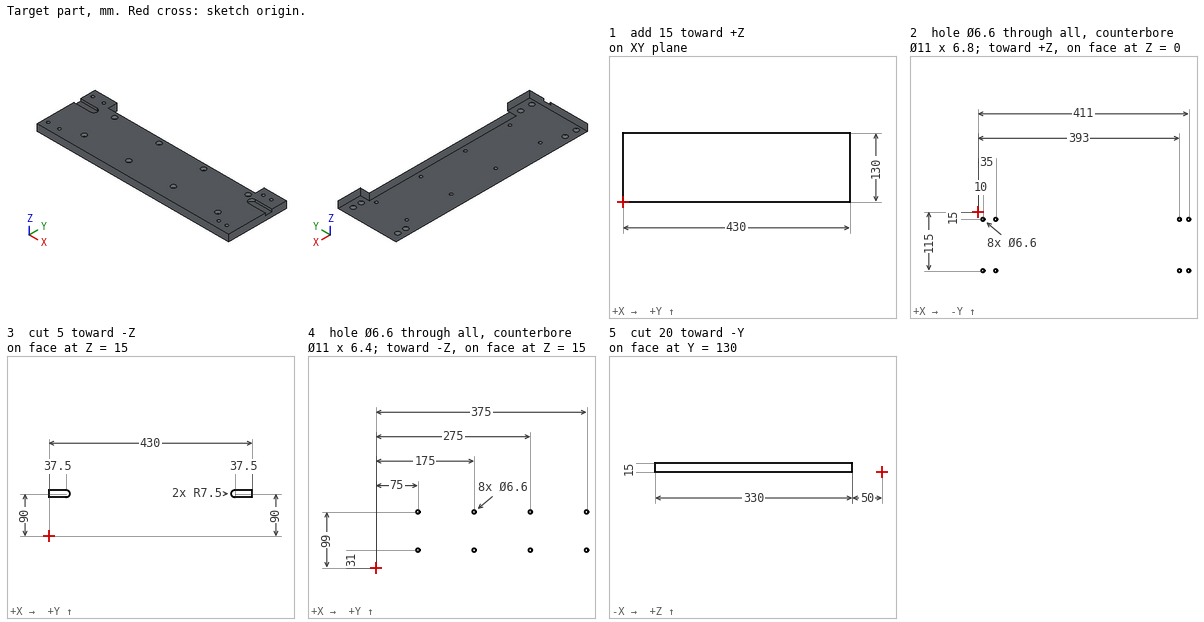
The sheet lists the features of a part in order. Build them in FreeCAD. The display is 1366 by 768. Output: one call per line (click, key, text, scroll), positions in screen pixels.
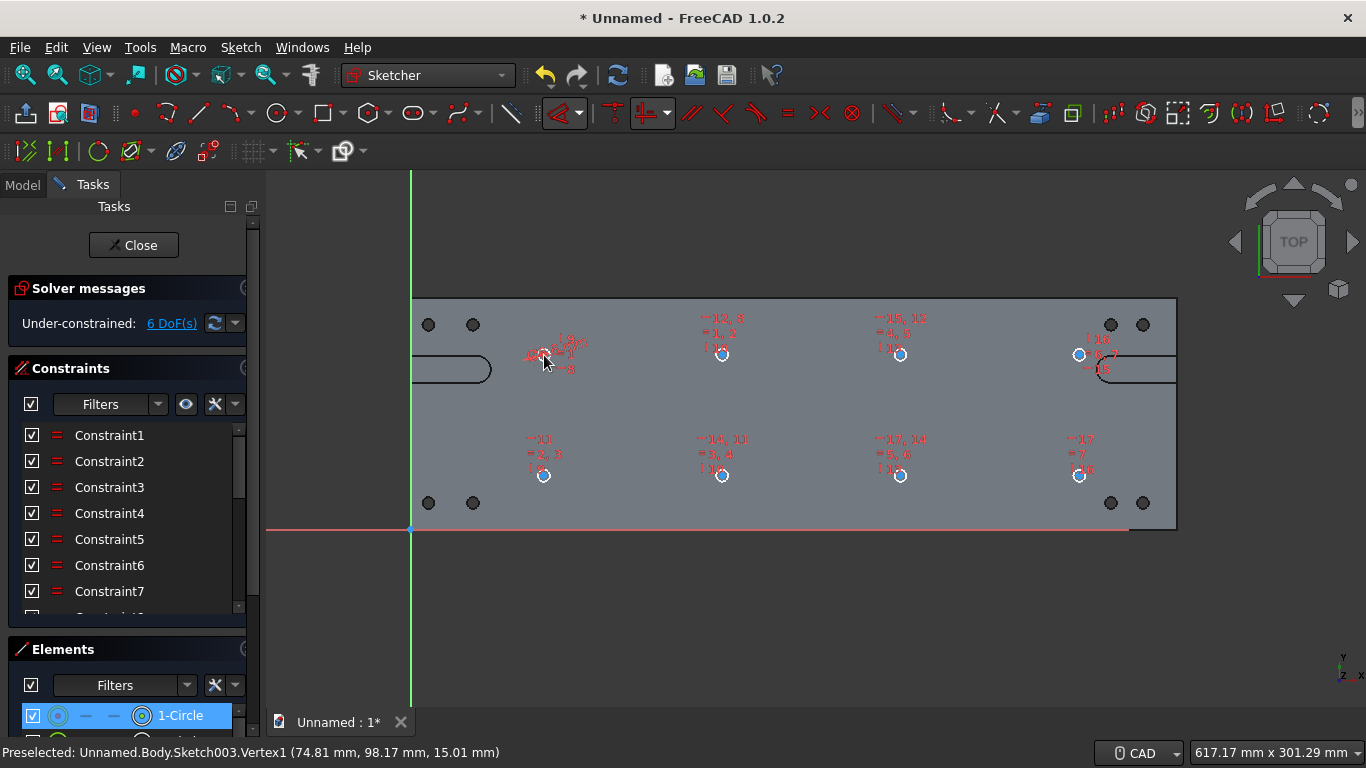
click(582, 114)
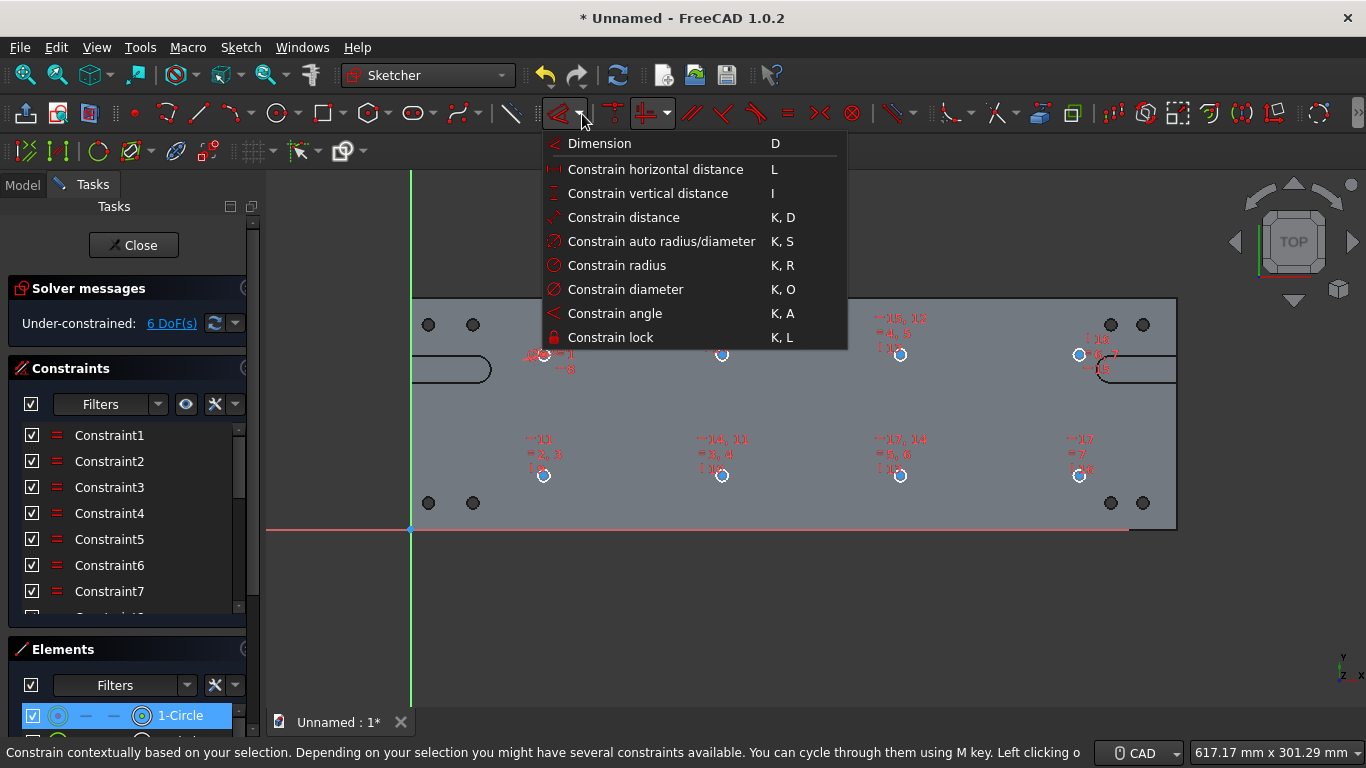
click(695, 169)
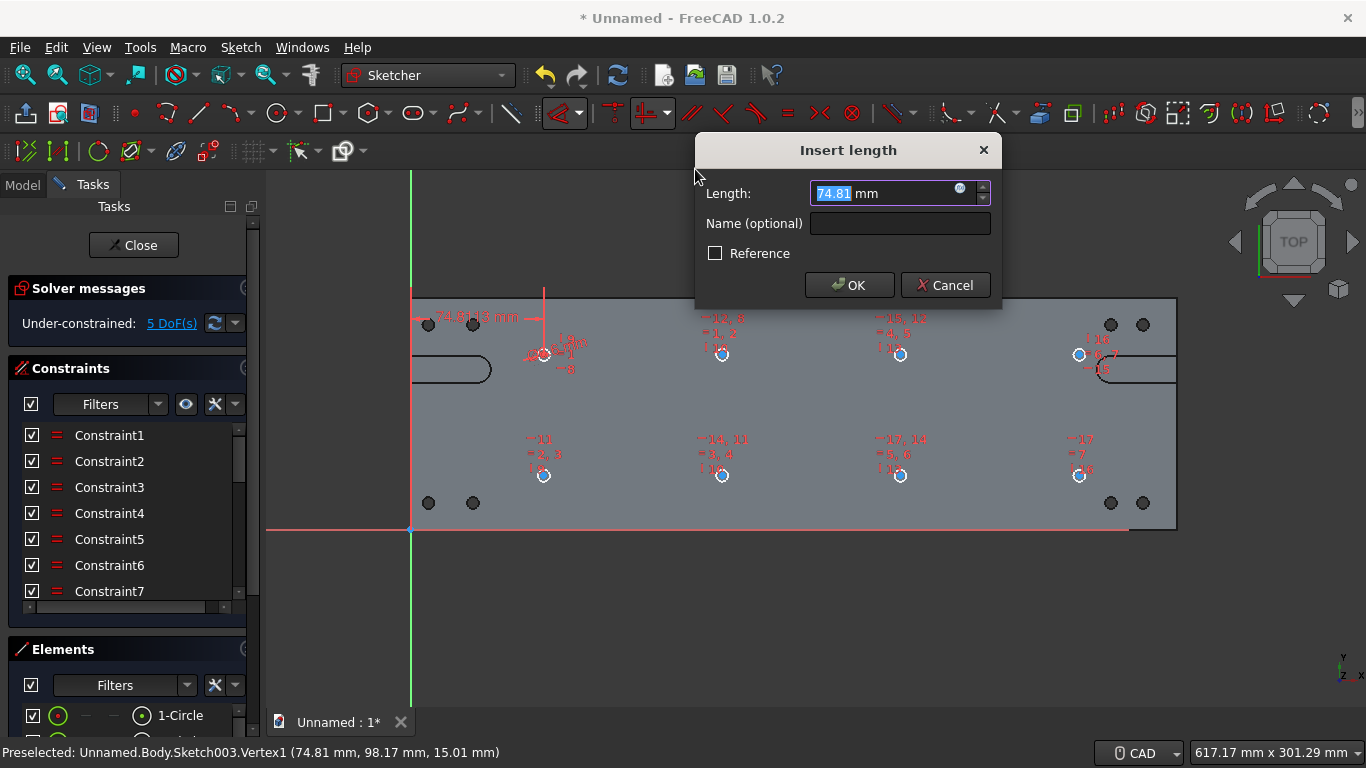
text(75)
key(Return)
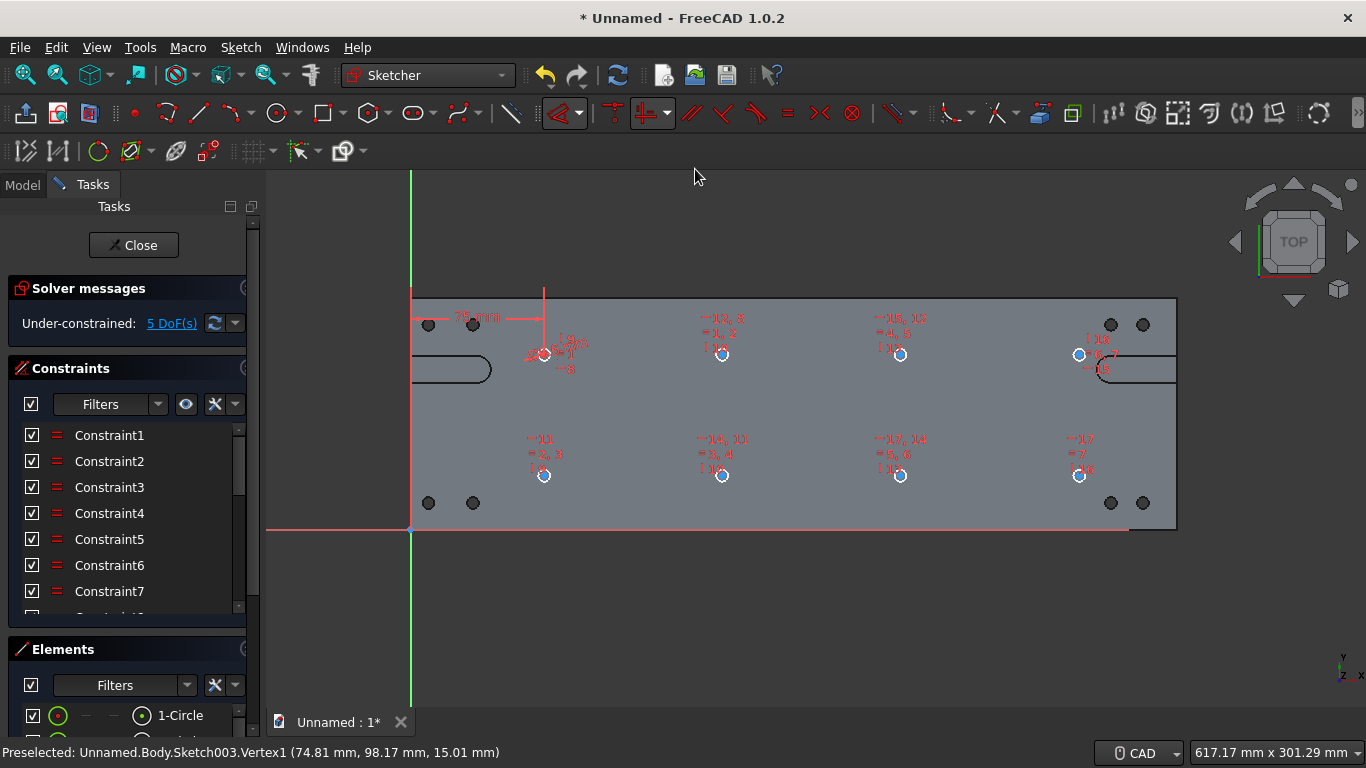
click(544, 355)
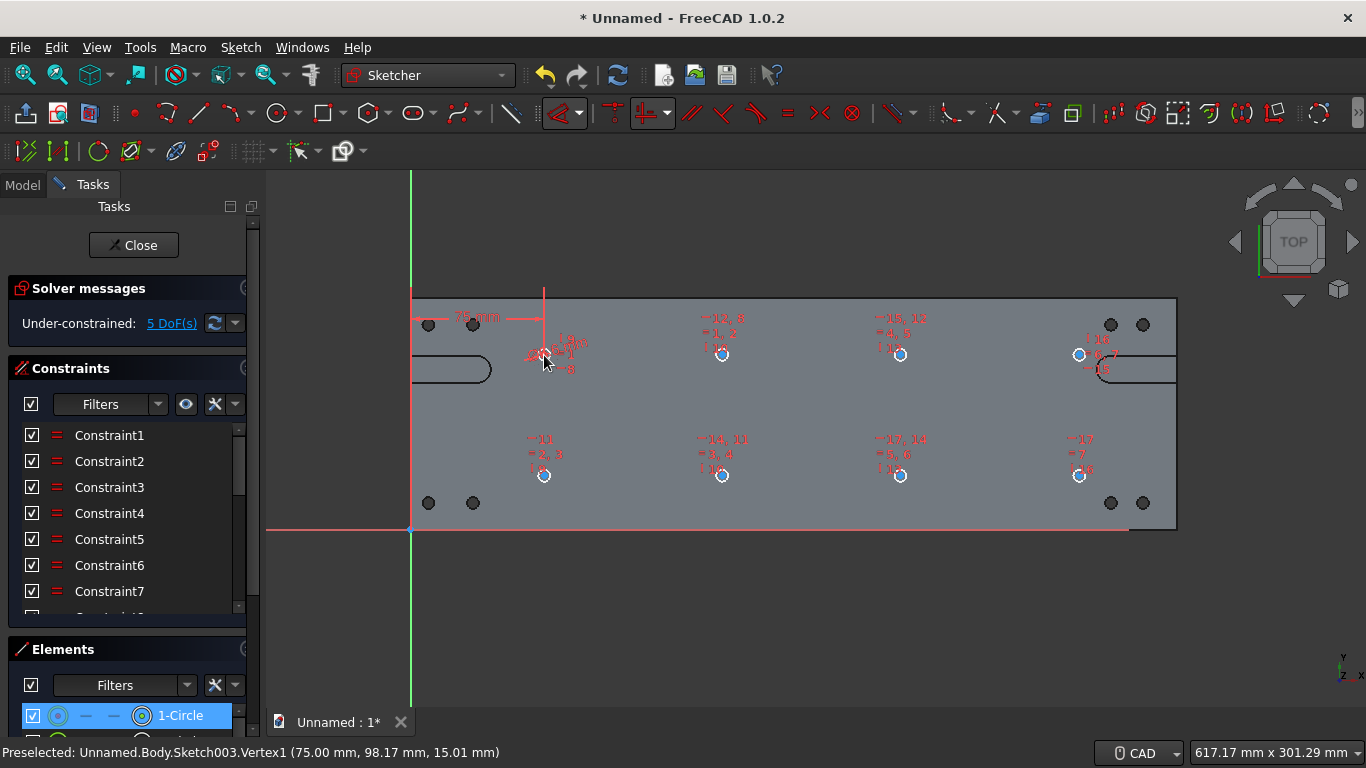
click(582, 114)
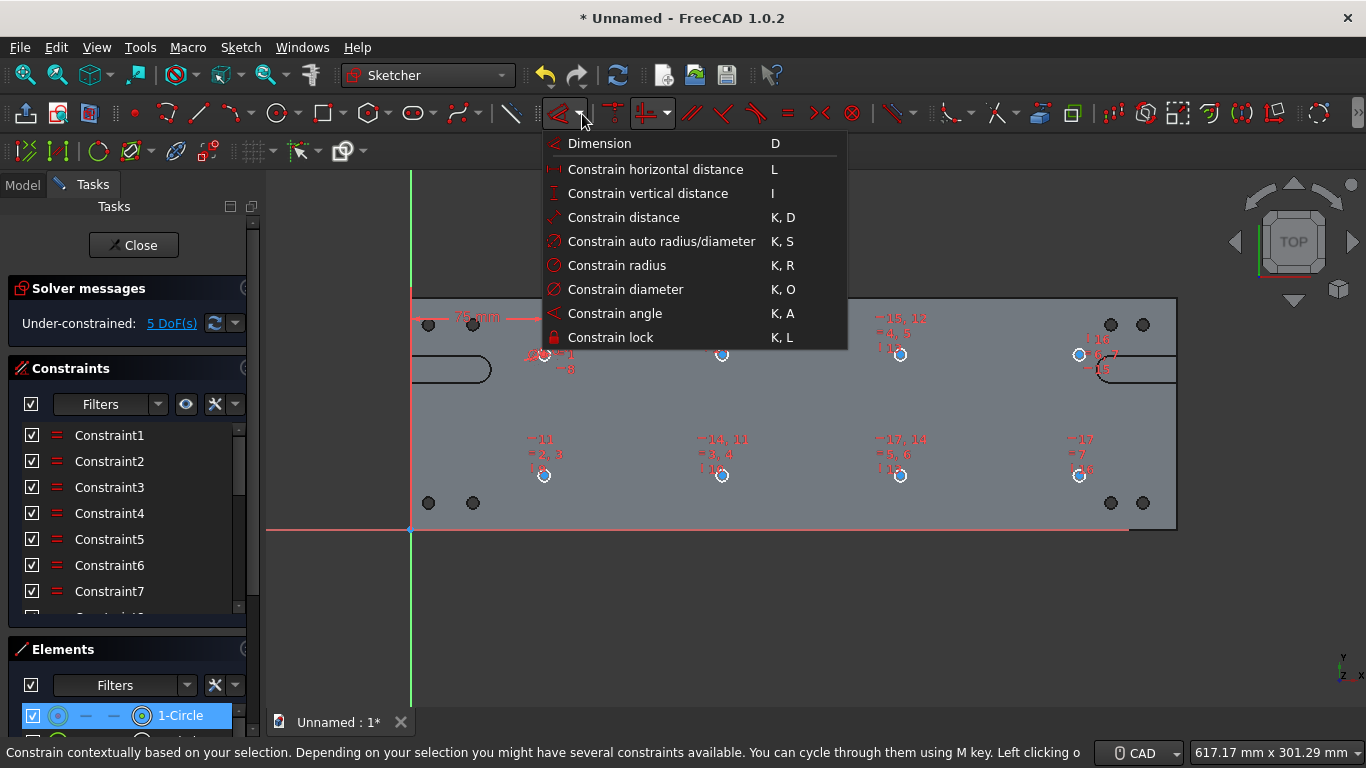
click(695, 193)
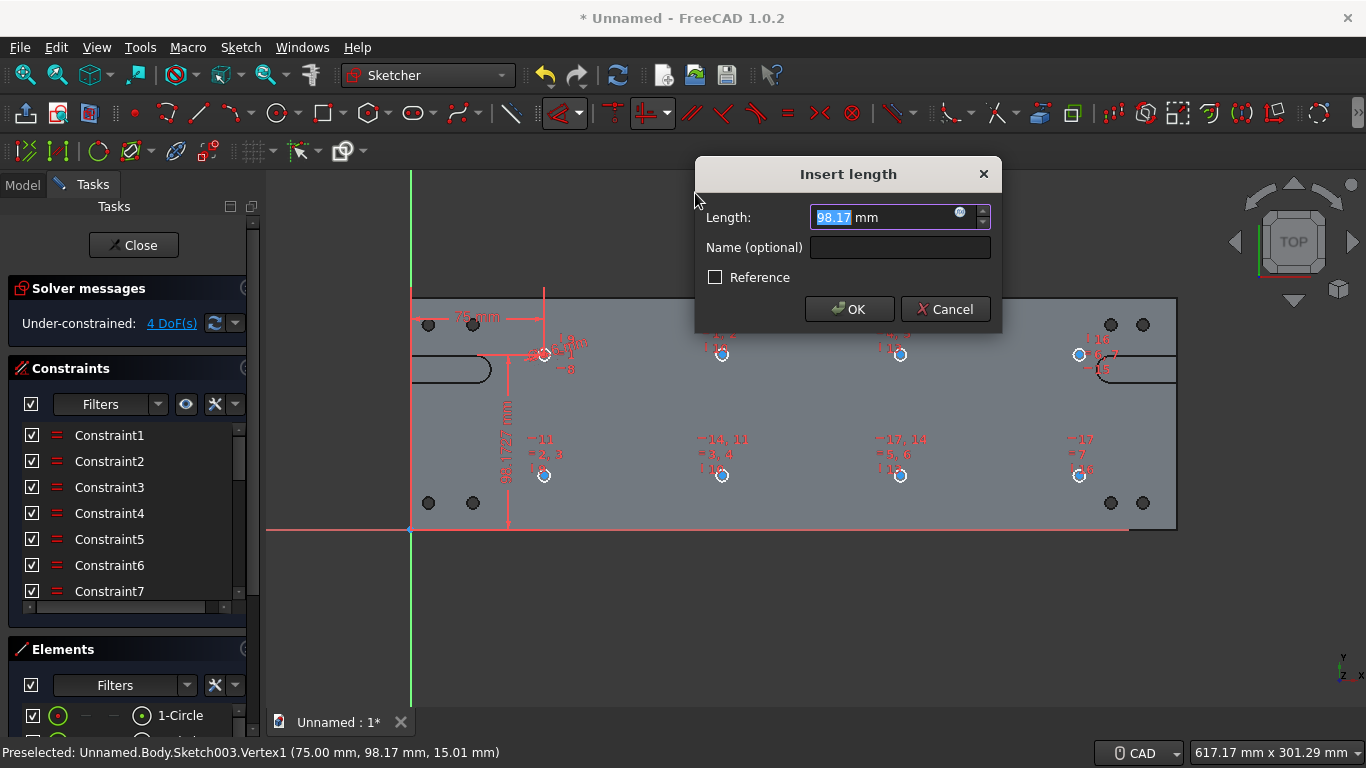
text(99)
key(Return)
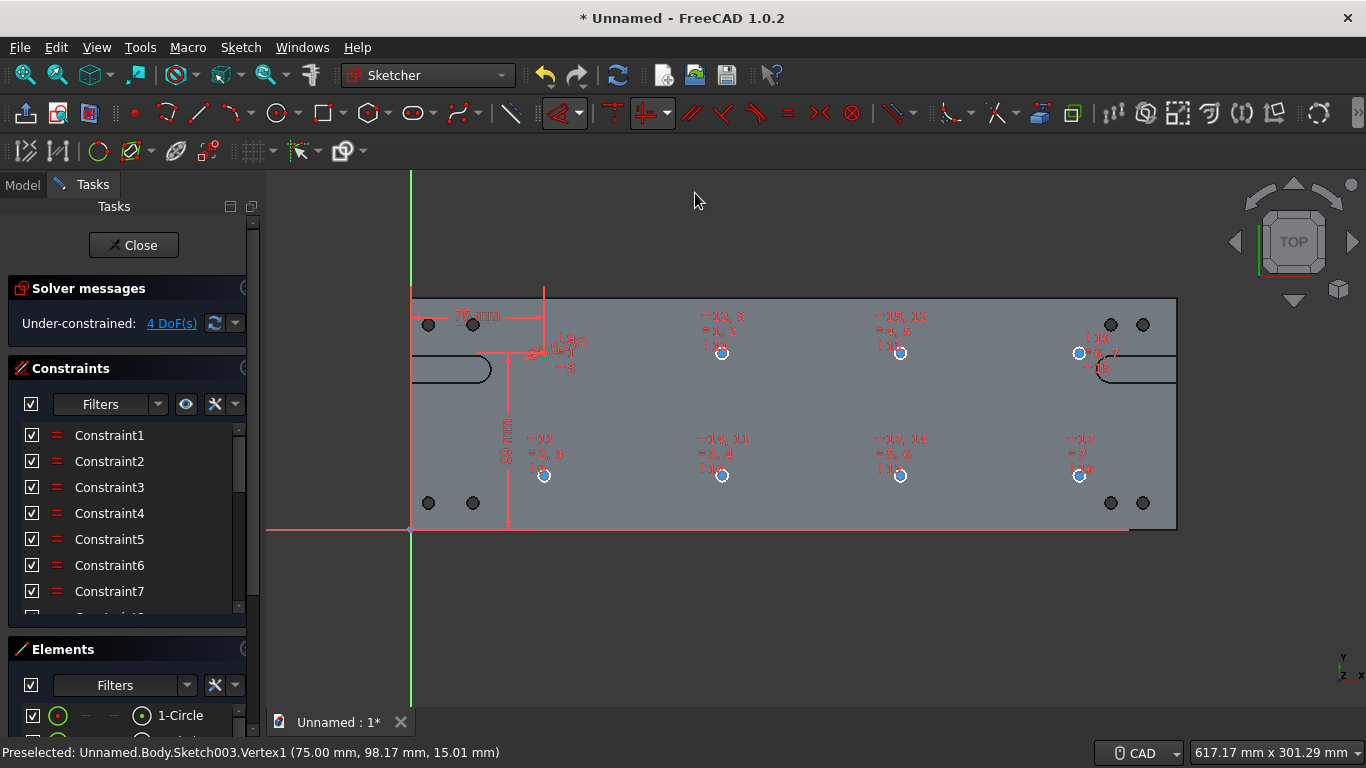
click(544, 476)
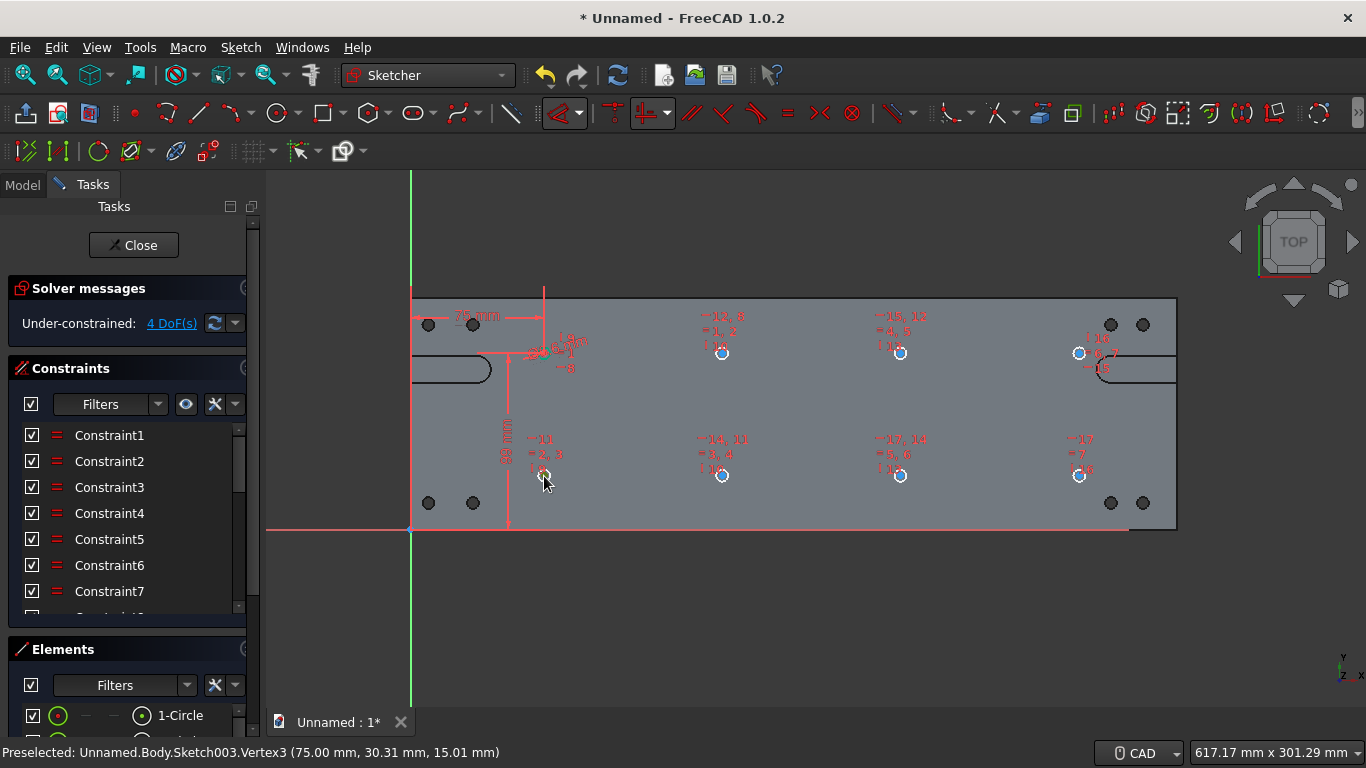
key(i)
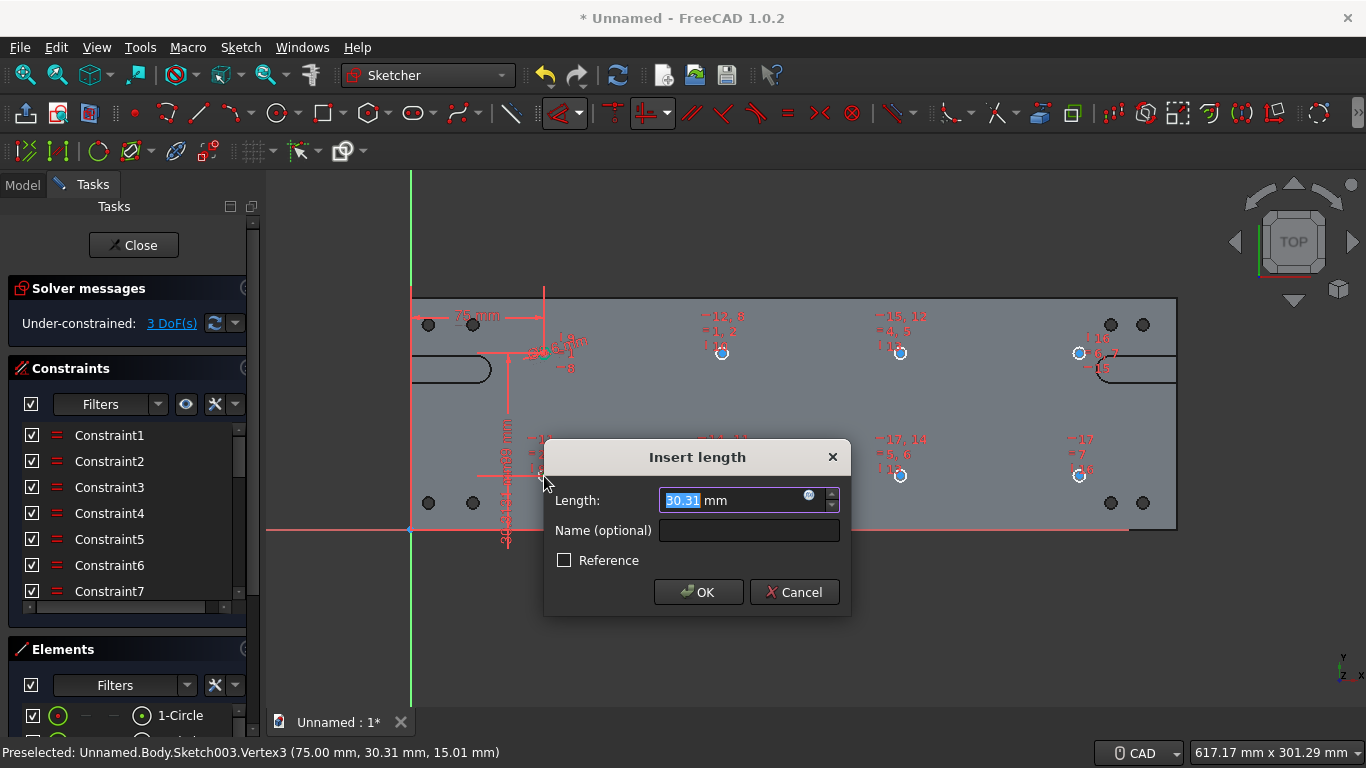
text(31)
key(Return)